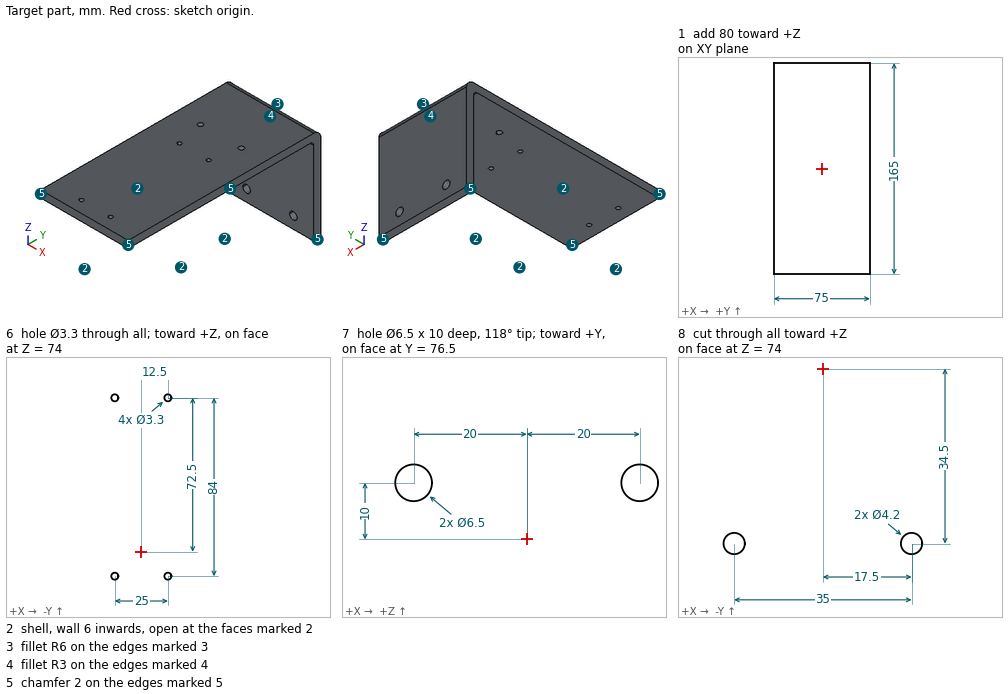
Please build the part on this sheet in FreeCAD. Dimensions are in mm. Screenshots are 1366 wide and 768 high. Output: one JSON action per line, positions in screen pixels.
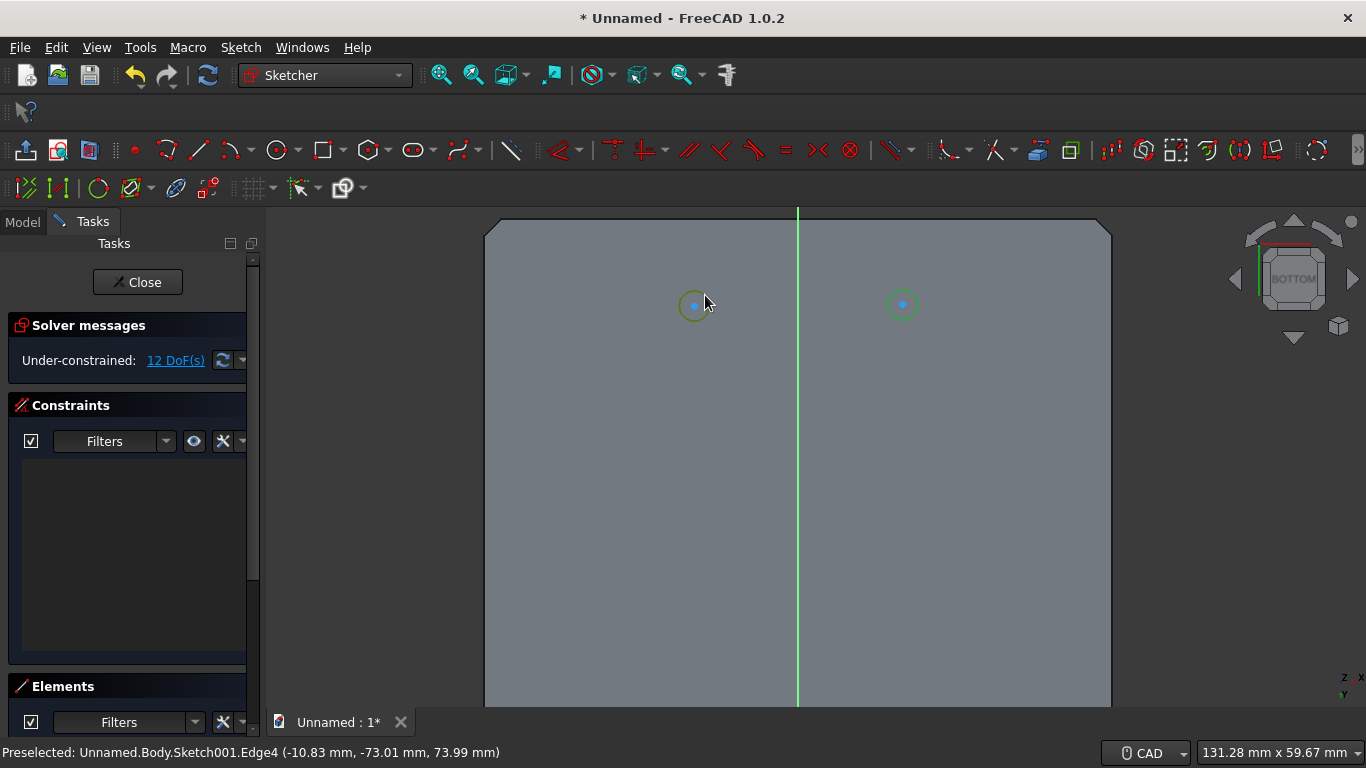
{"action": "left_click", "coordinate": [786, 150]}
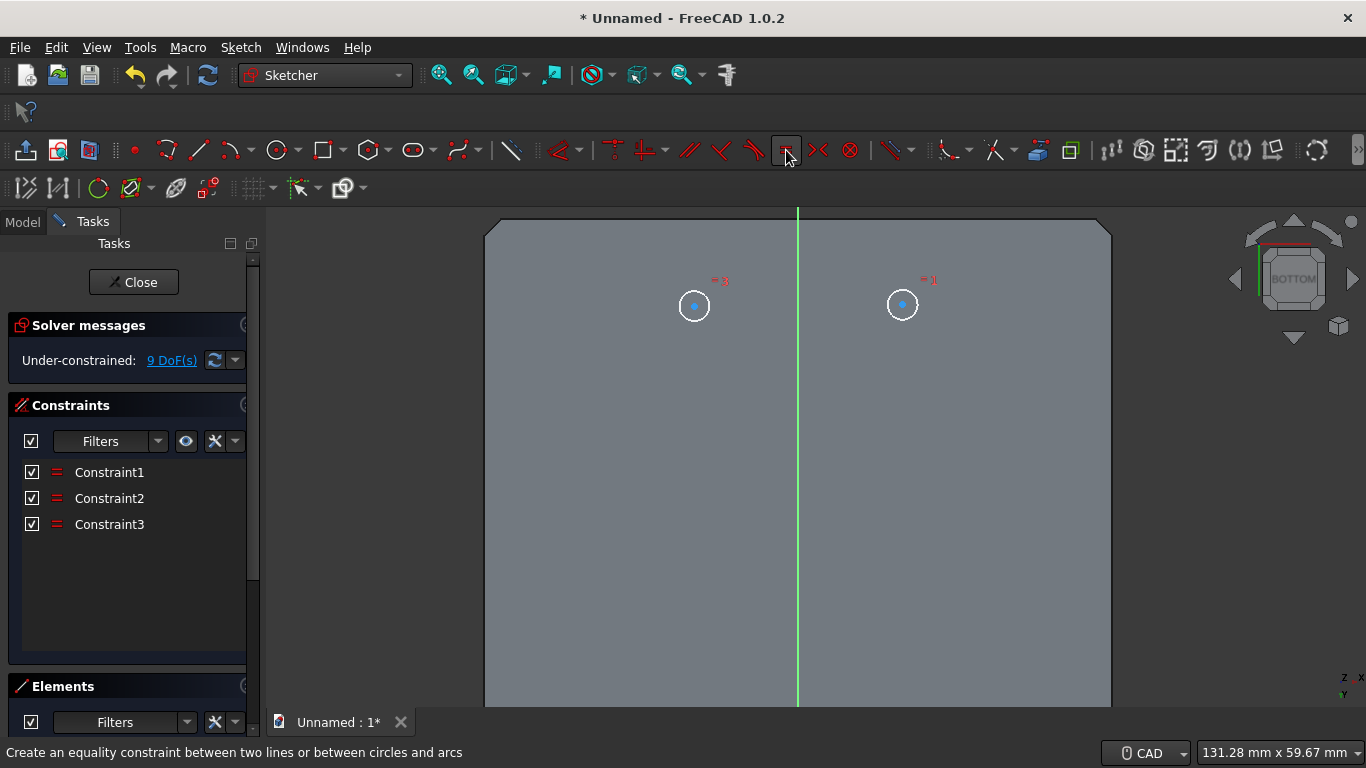
{"action": "left_click", "coordinate": [903, 305]}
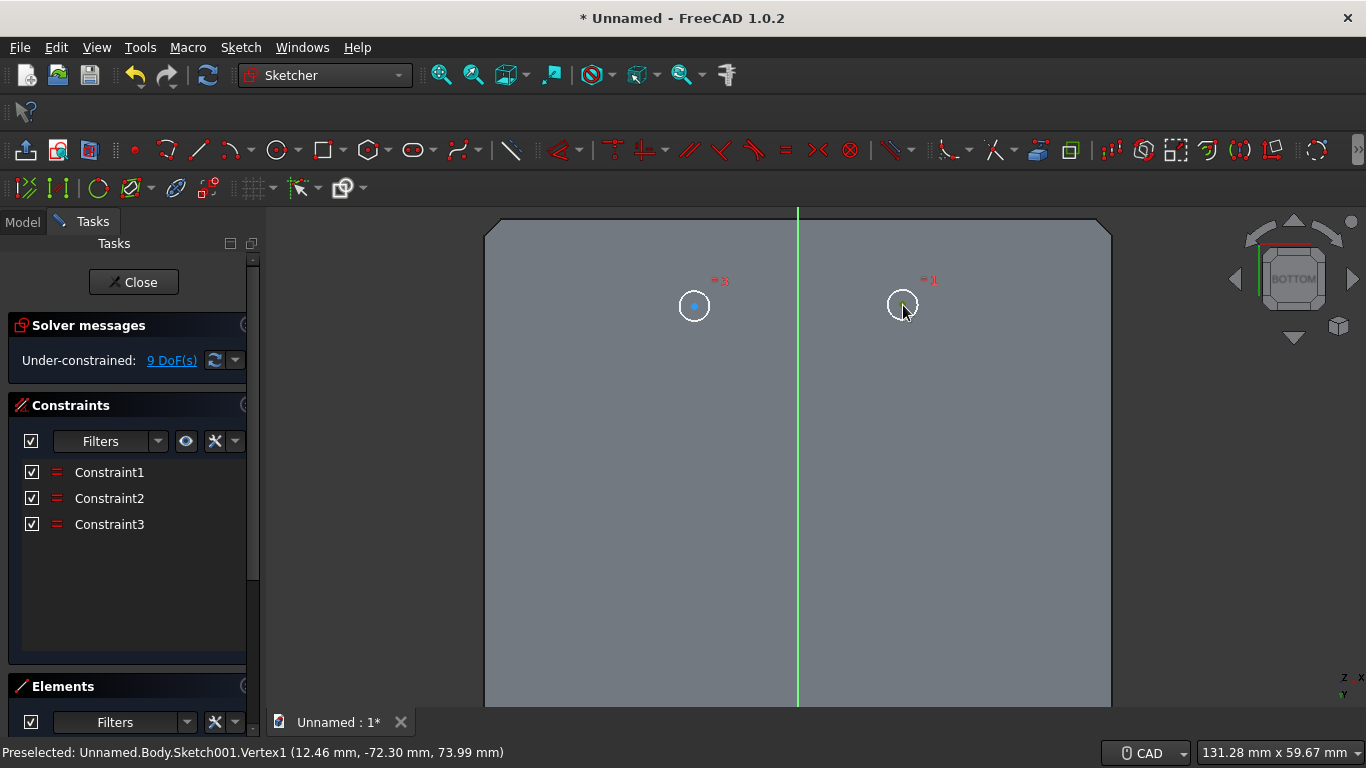
{"action": "scroll", "coordinate": [706, 295], "scroll_direction": "down", "scroll_amount": 4}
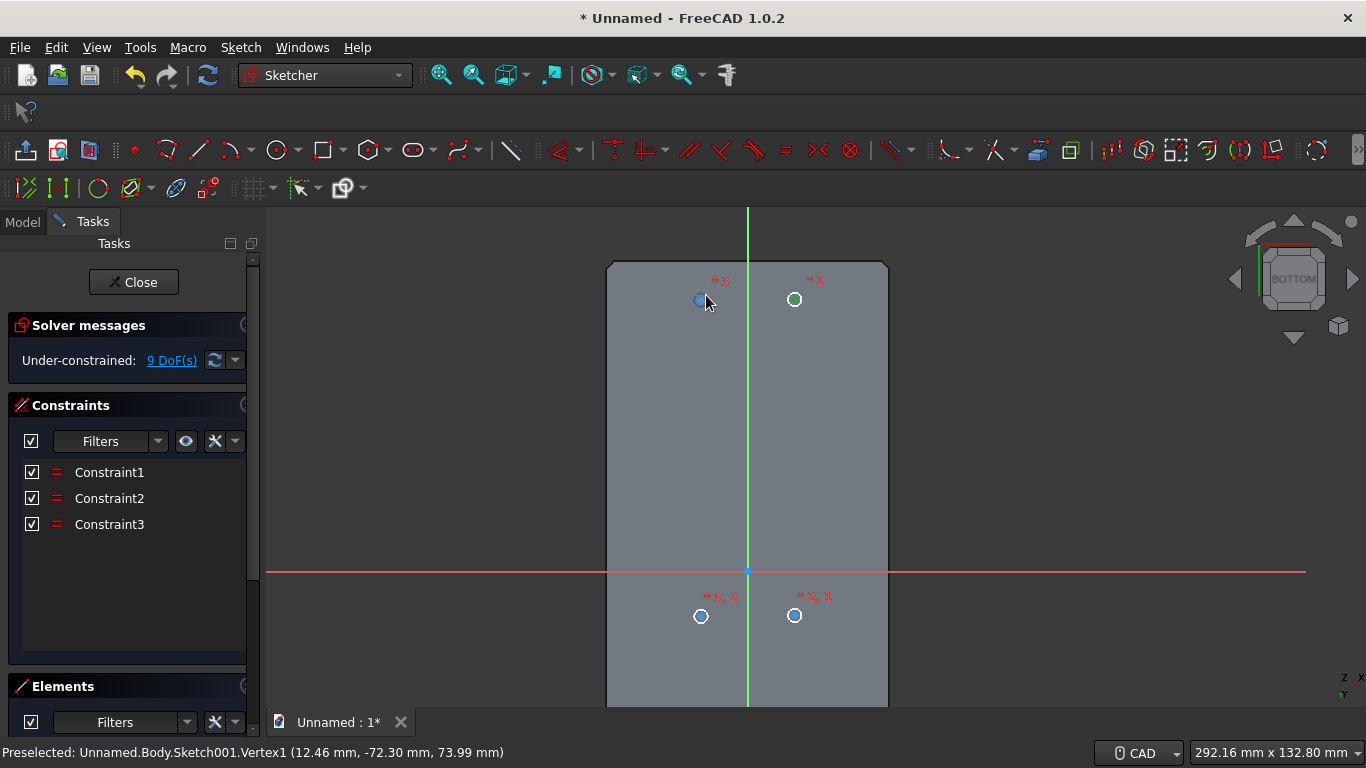
{"action": "left_click", "coordinate": [795, 615]}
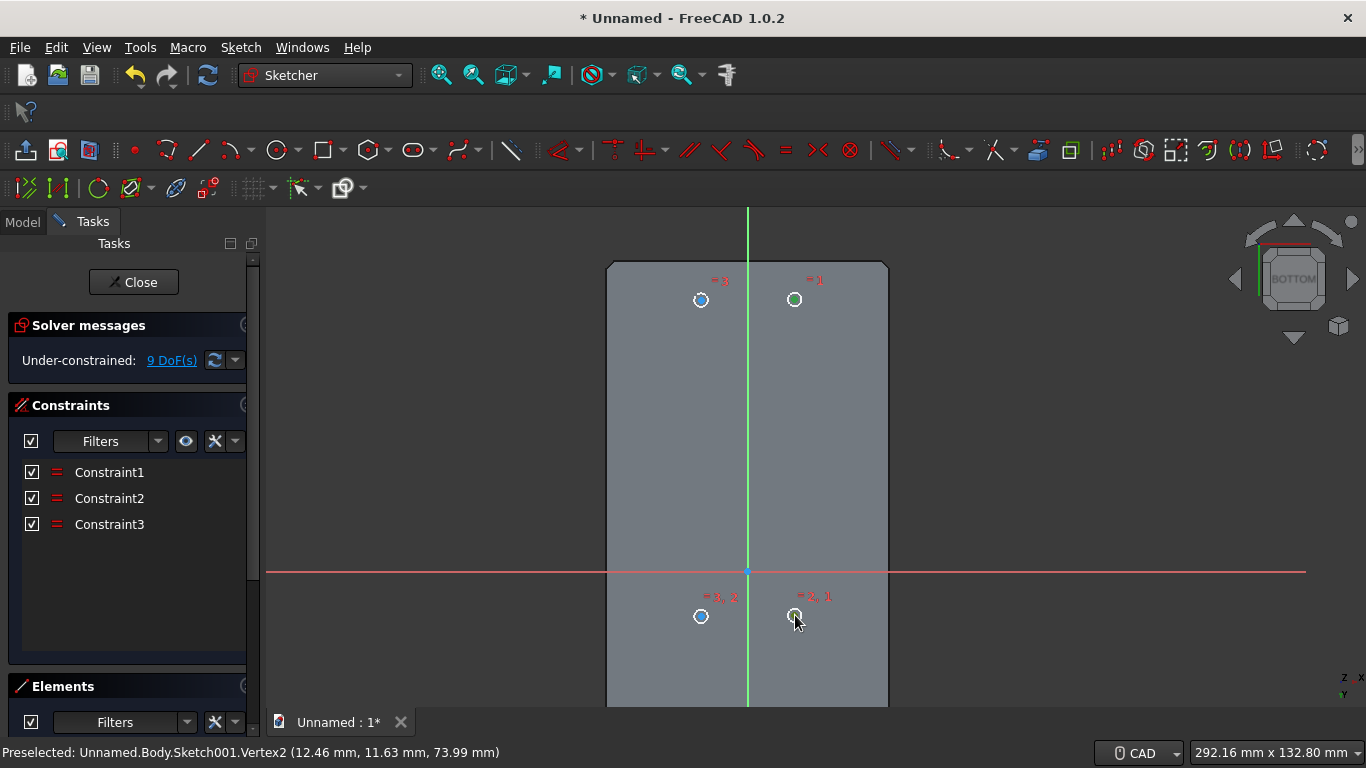
{"action": "key", "text": "v"}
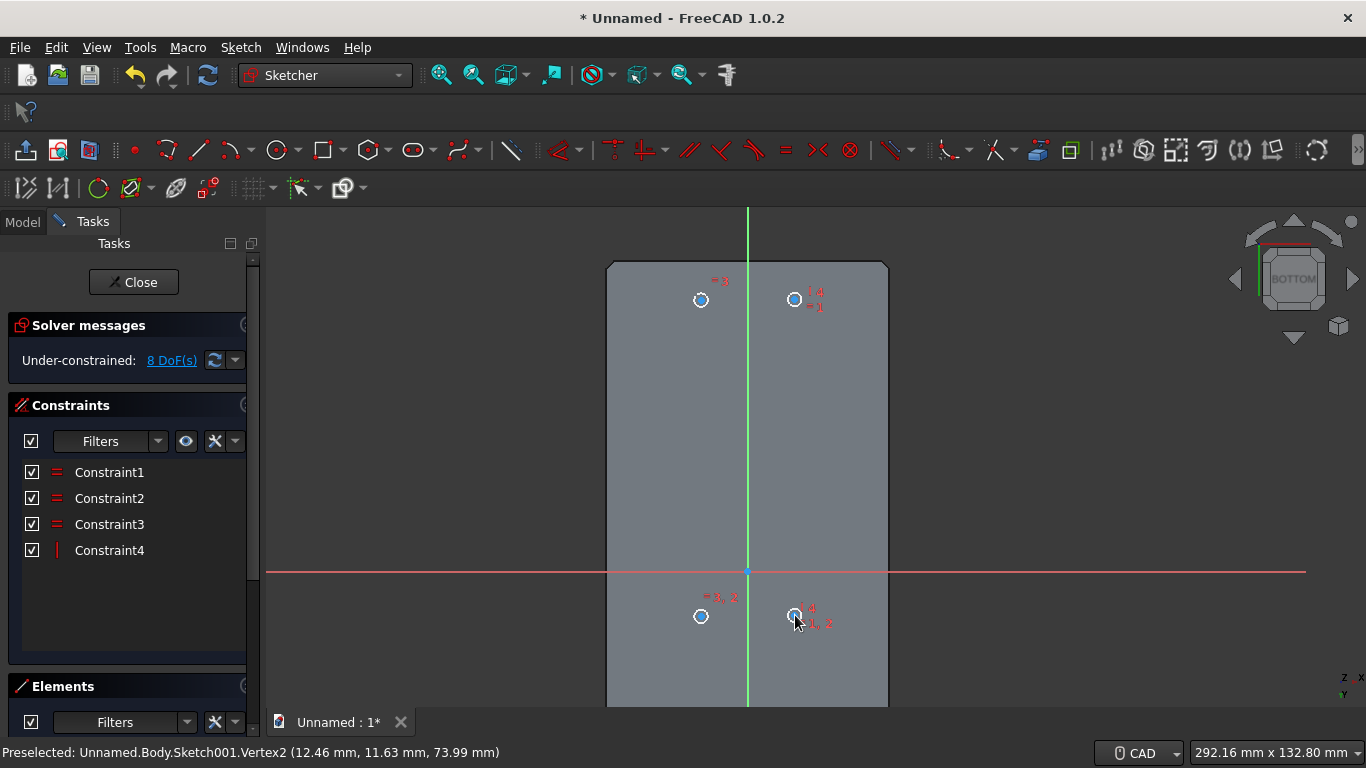
{"action": "left_click", "coordinate": [795, 615]}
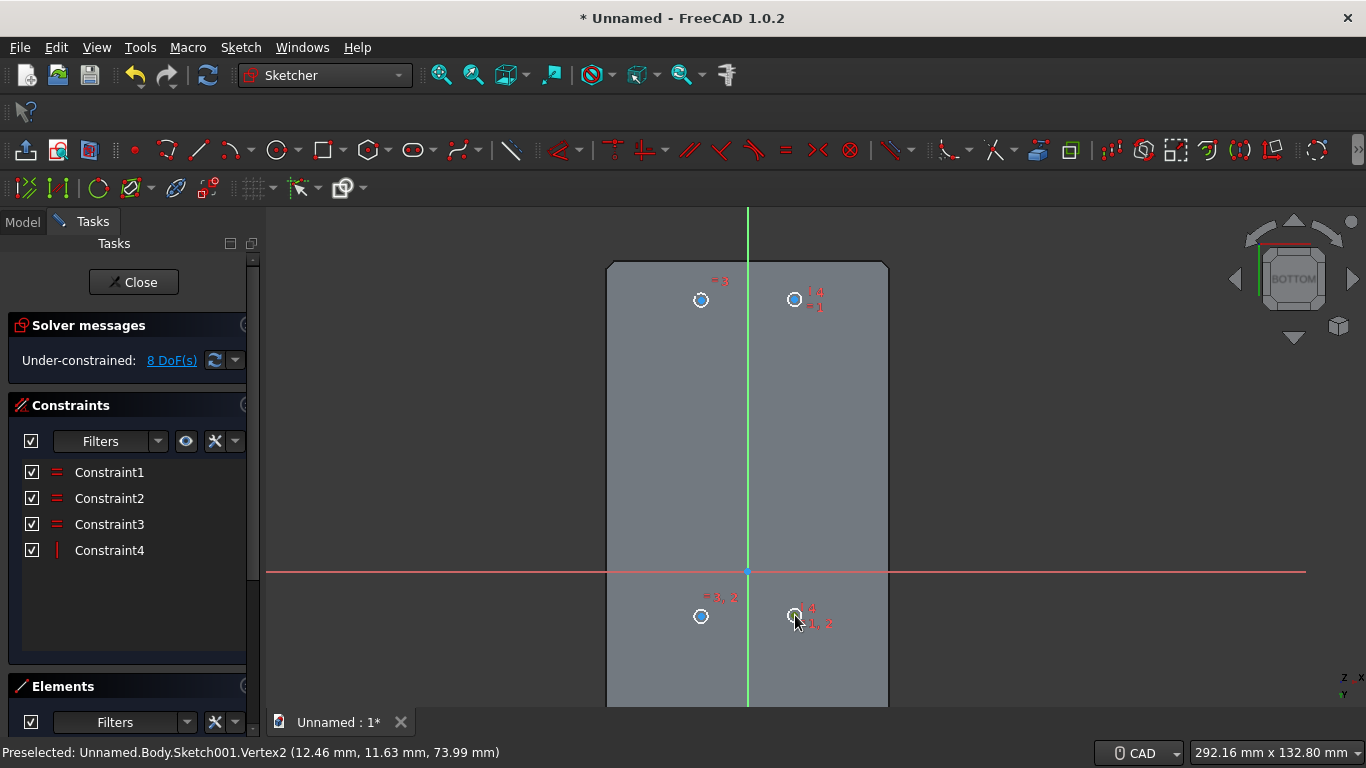
{"action": "left_click", "coordinate": [701, 616]}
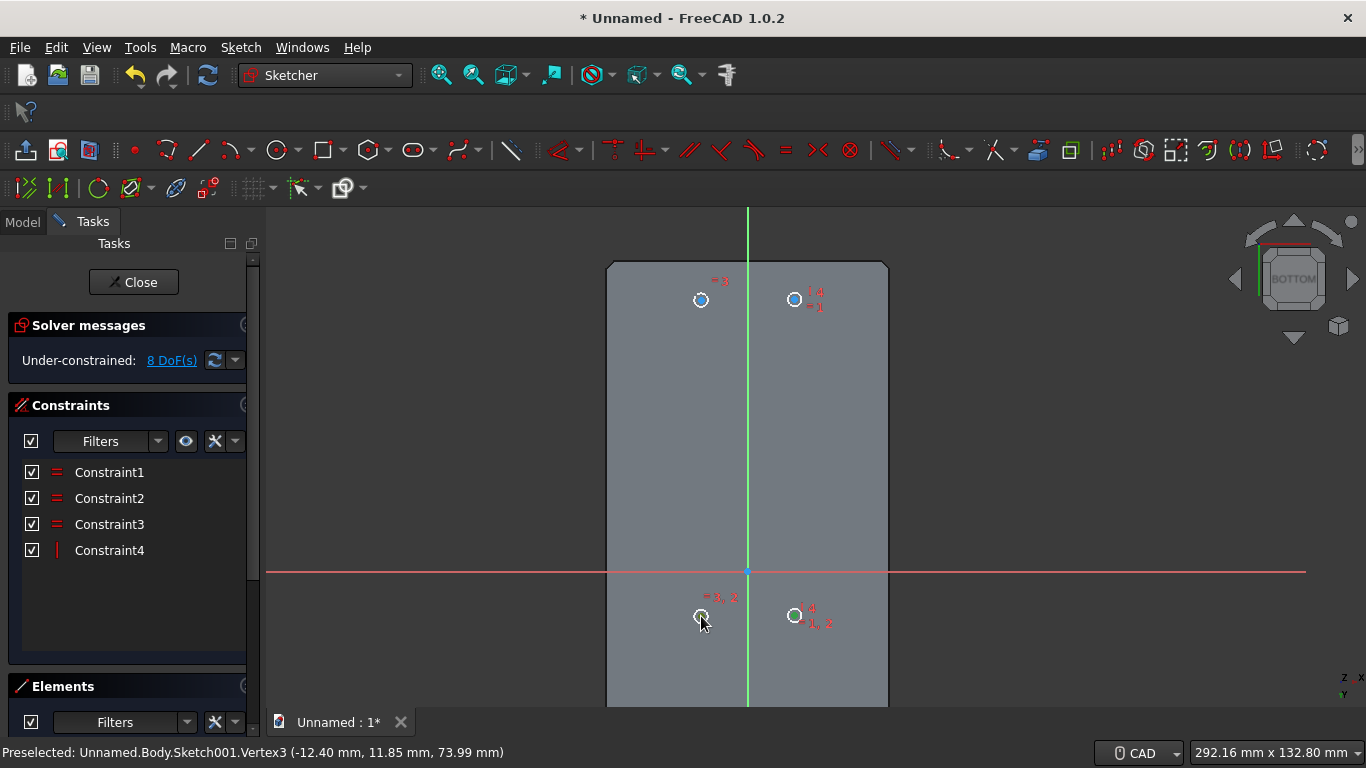
{"action": "left_click", "coordinate": [668, 150]}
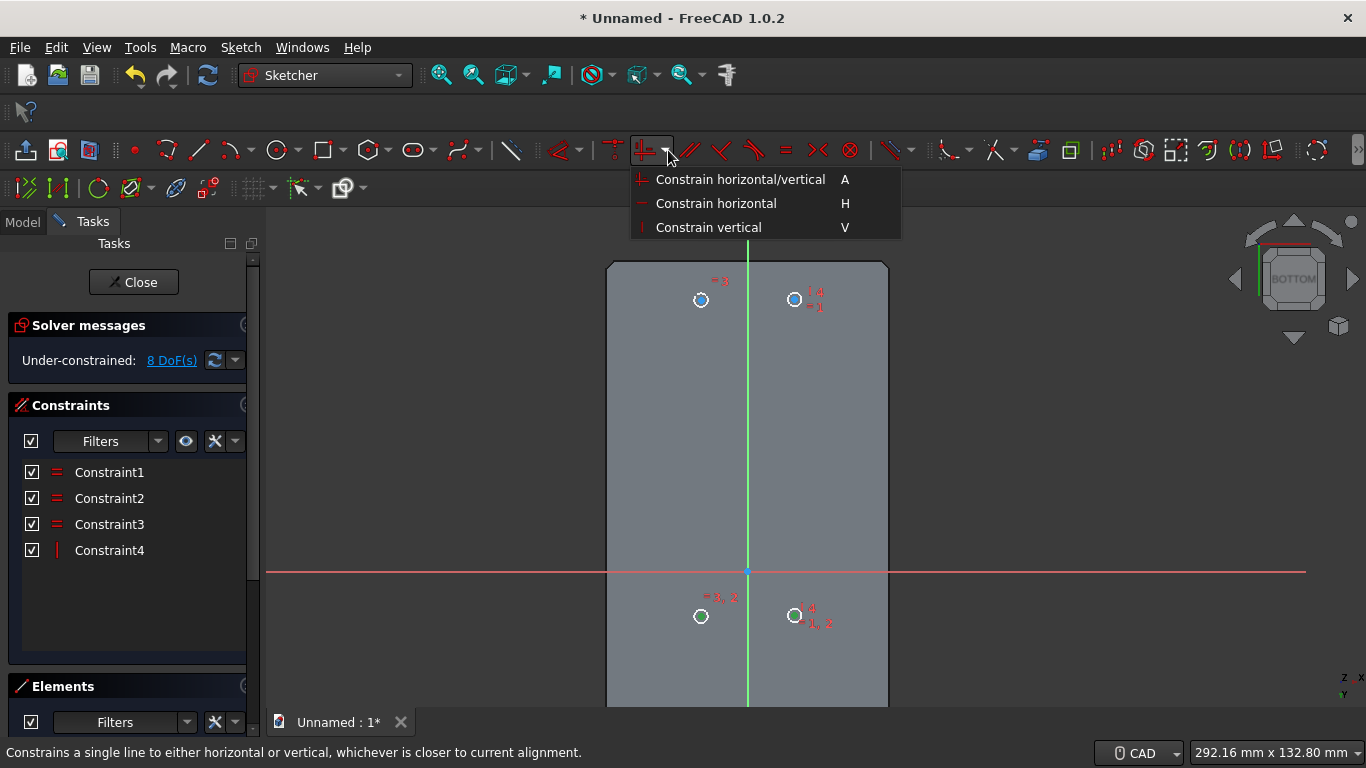
{"action": "left_click", "coordinate": [766, 203]}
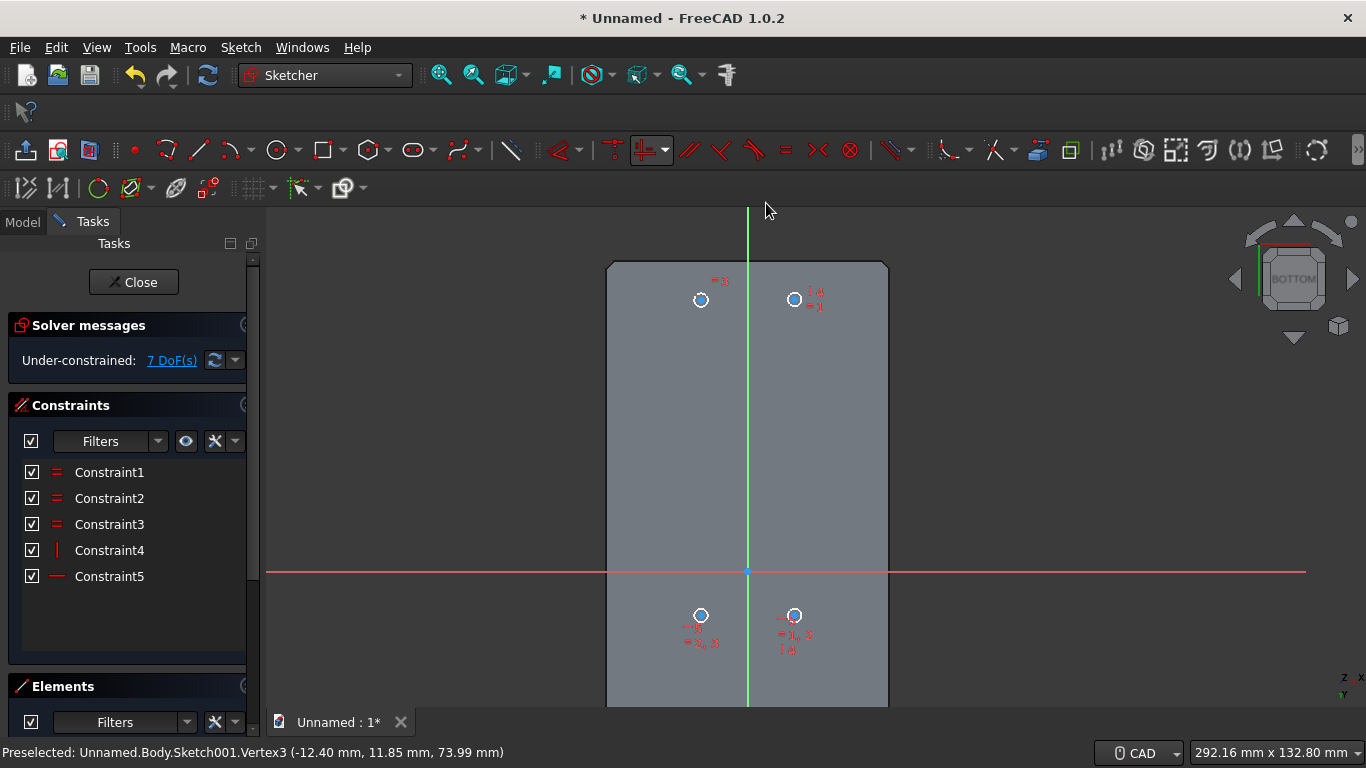
{"action": "left_click", "coordinate": [701, 615]}